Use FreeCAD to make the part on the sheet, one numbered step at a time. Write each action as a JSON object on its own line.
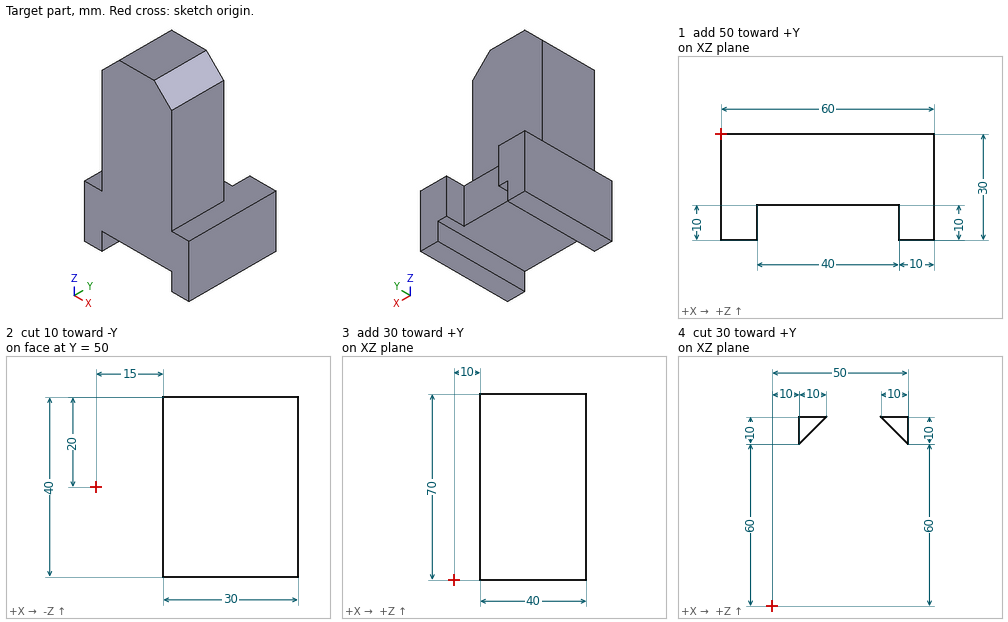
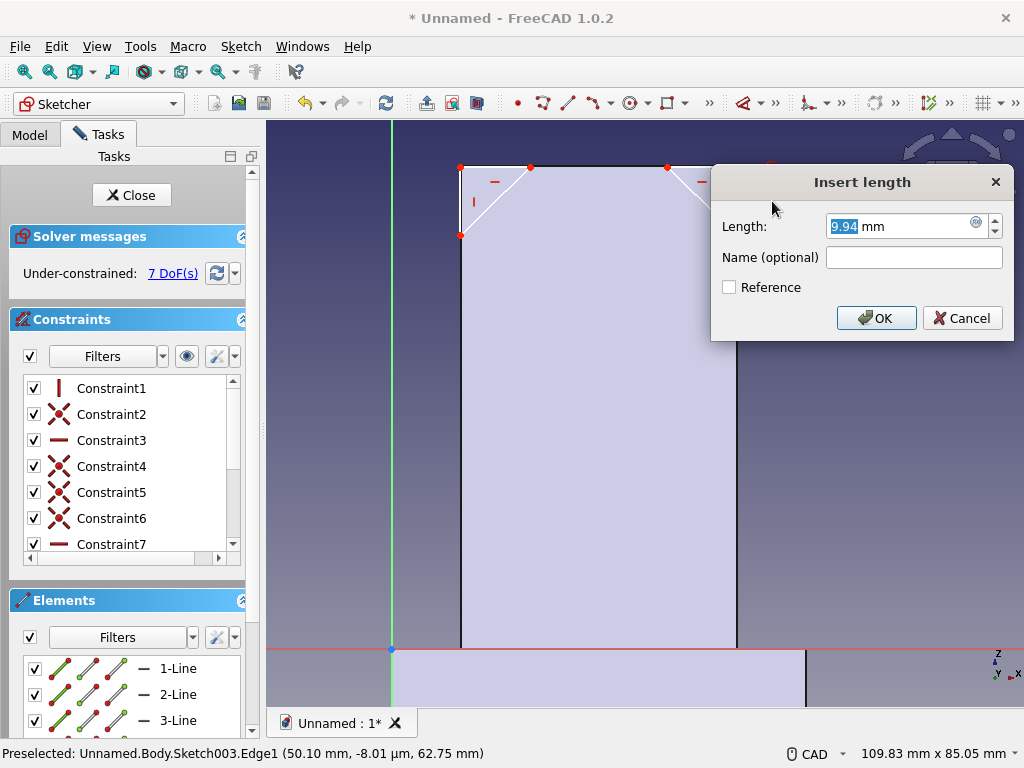
{"action": "type", "text": "10"}
{"action": "key", "text": "Return"}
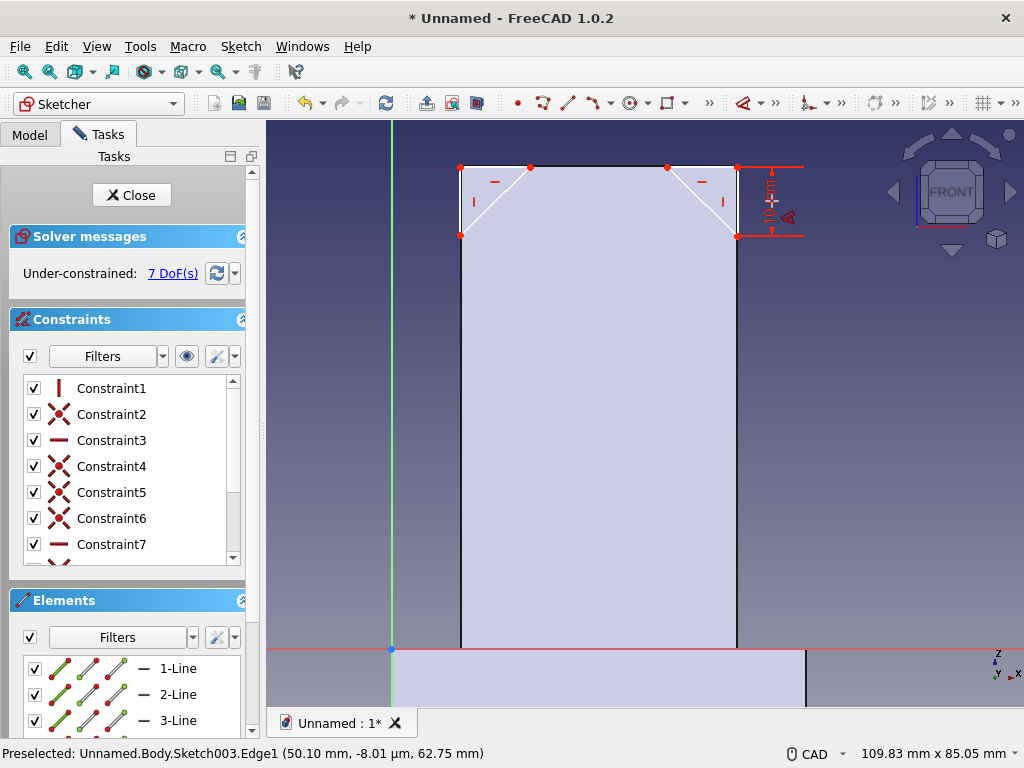
{"action": "left_click", "coordinate": [717, 167]}
{"action": "left_click", "coordinate": [678, 201]}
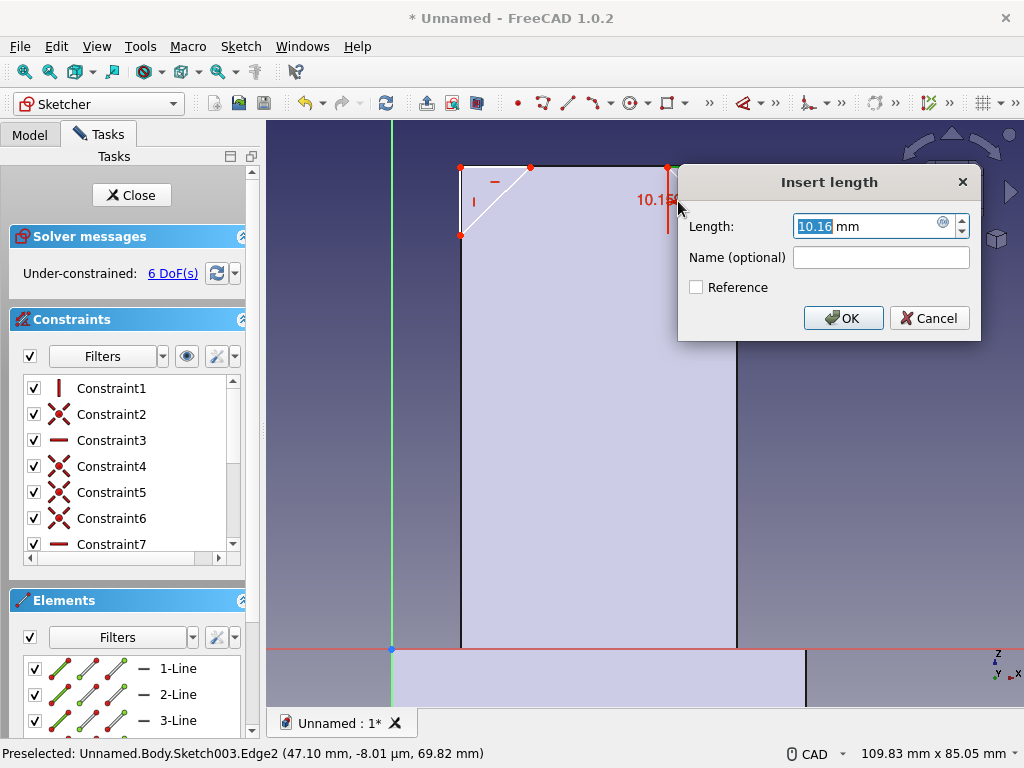
{"action": "type", "text": "10"}
{"action": "key", "text": "Return"}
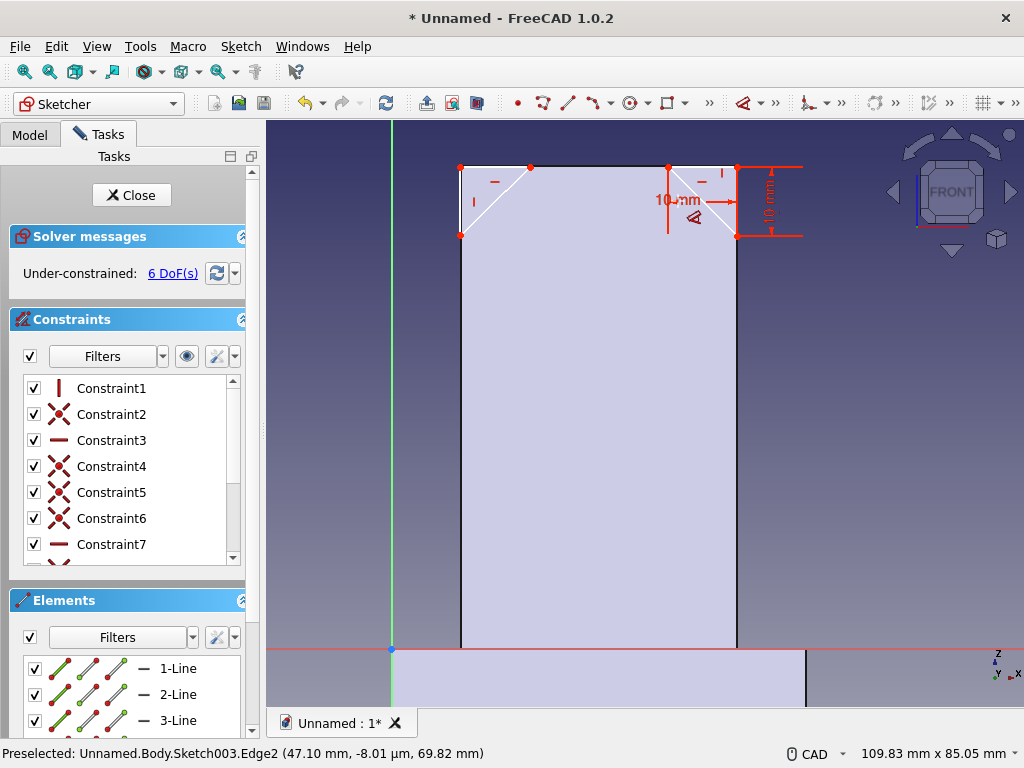
{"action": "left_click", "coordinate": [509, 167]}
{"action": "left_click", "coordinate": [520, 201]}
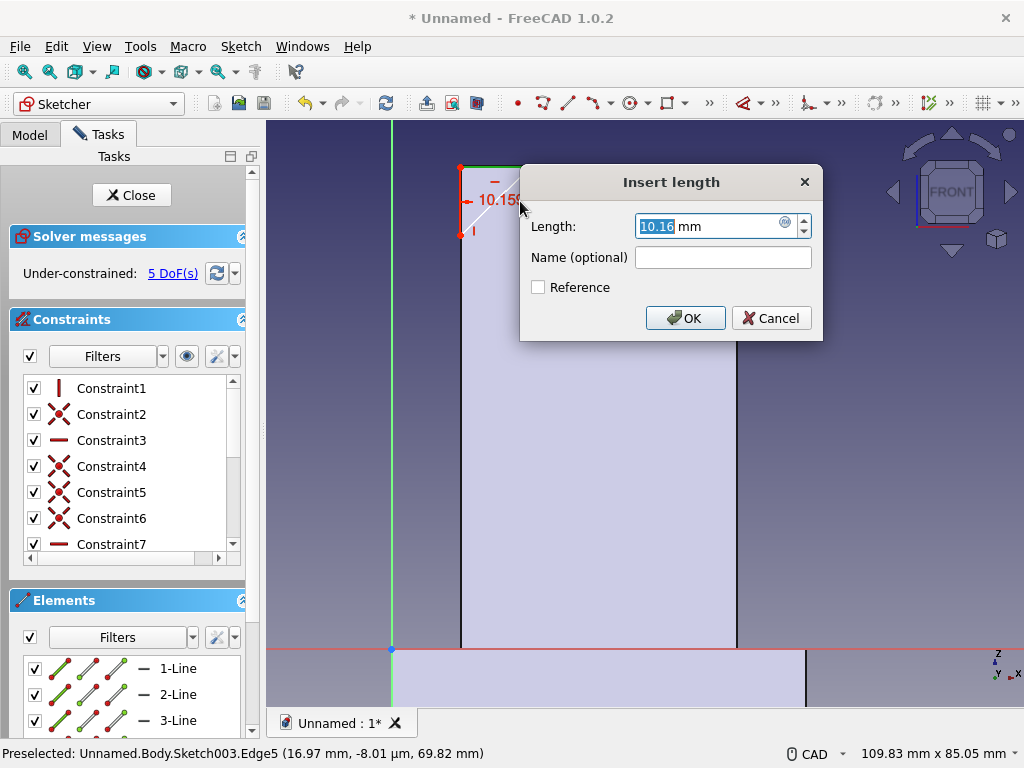
{"action": "type", "text": "10"}
{"action": "key", "text": "Return"}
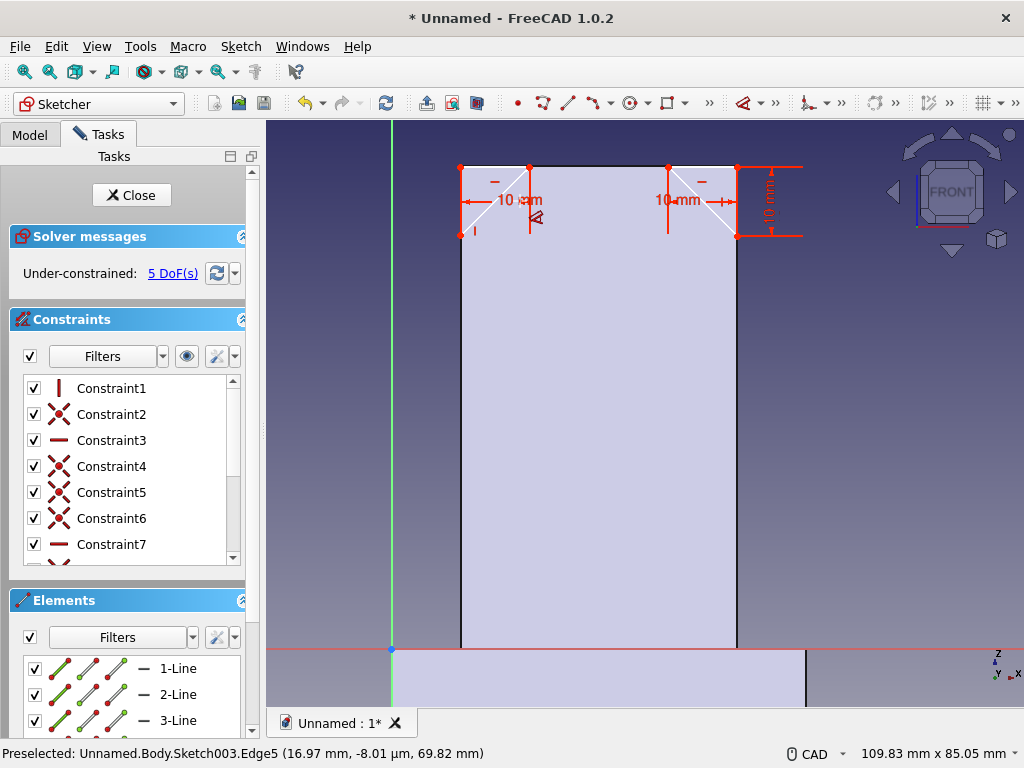
{"action": "left_click", "coordinate": [461, 188]}
{"action": "left_click", "coordinate": [427, 201]}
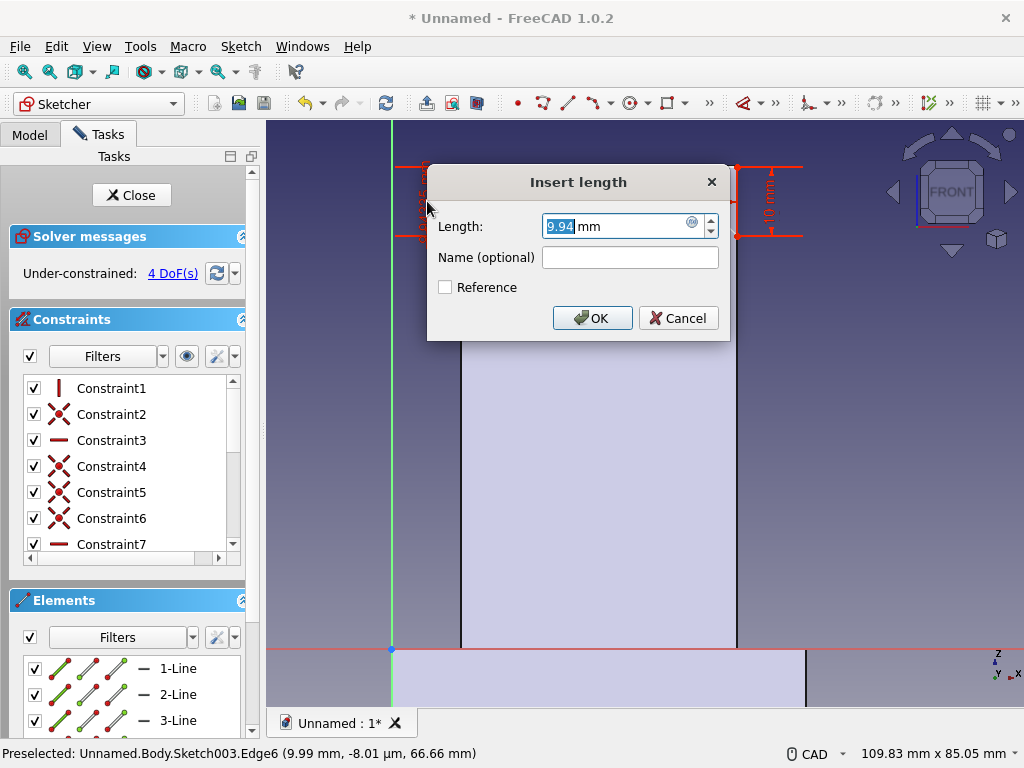
{"action": "type", "text": "10"}
{"action": "key", "text": "Return"}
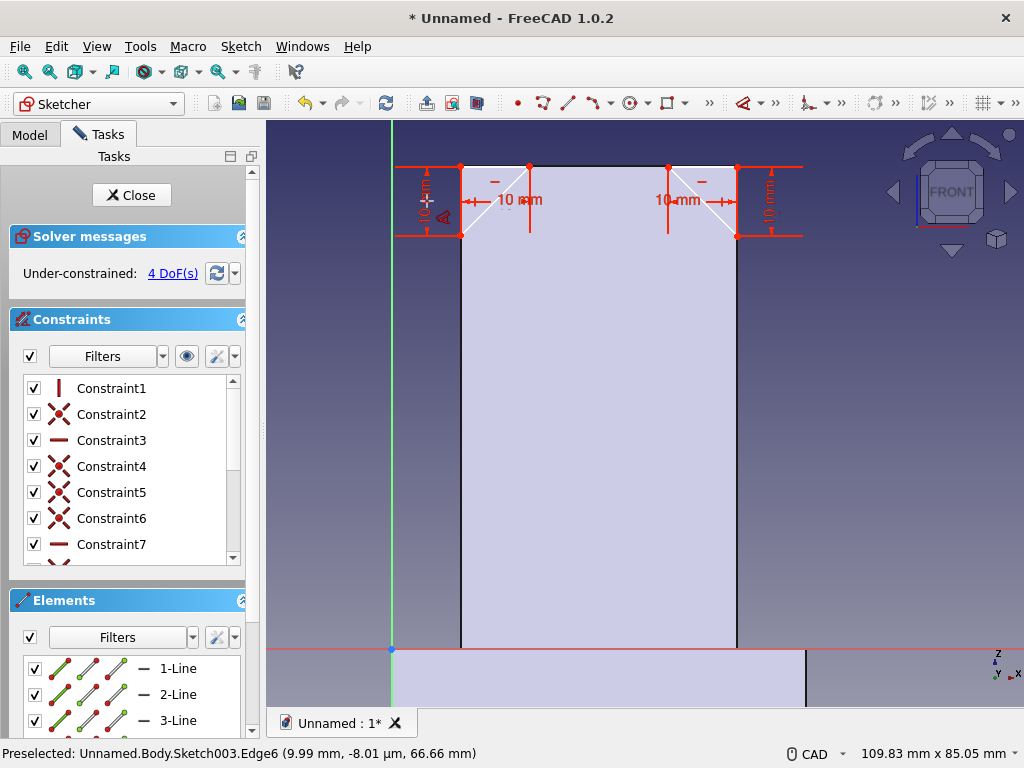
{"action": "left_click", "coordinate": [737, 236]}
{"action": "left_click", "coordinate": [565, 178]}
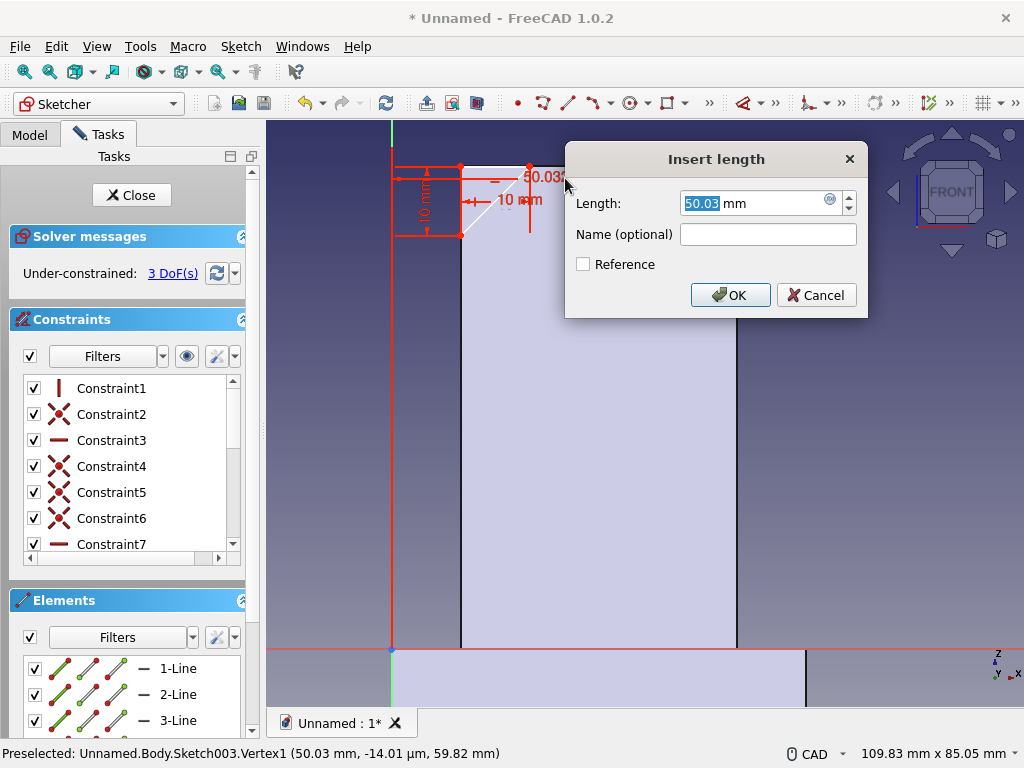
{"action": "type", "text": "50"}
{"action": "key", "text": "Return"}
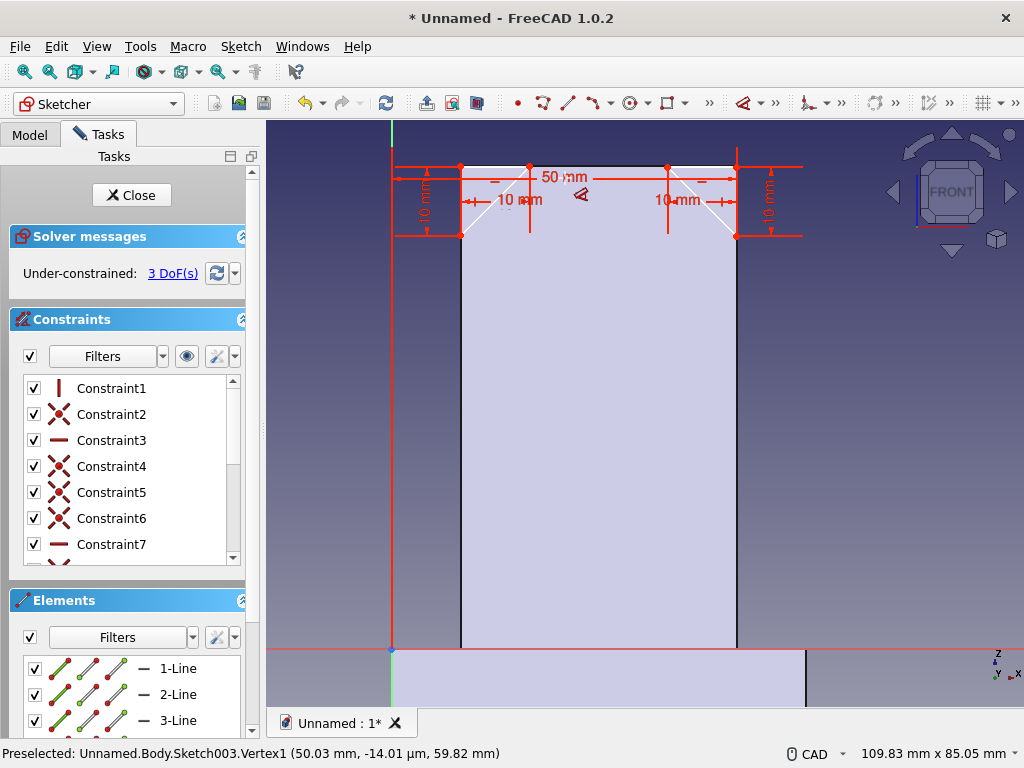
{"action": "left_click", "coordinate": [737, 236]}
{"action": "left_click", "coordinate": [771, 443]}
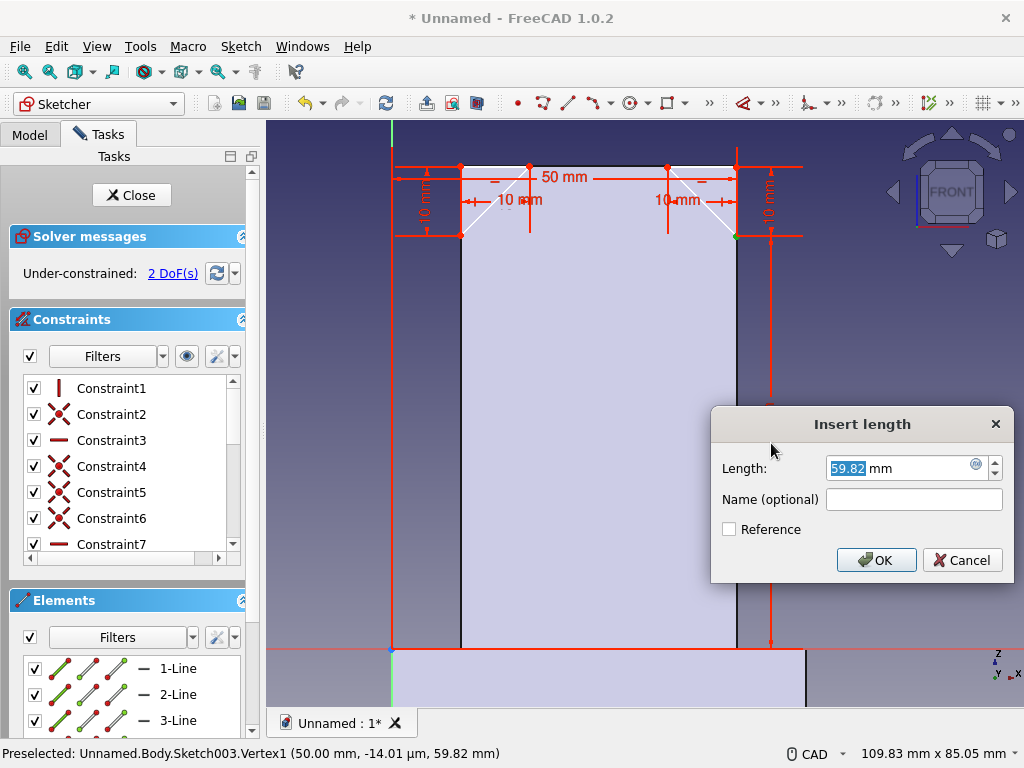
{"action": "type", "text": "60"}
{"action": "key", "text": "Return"}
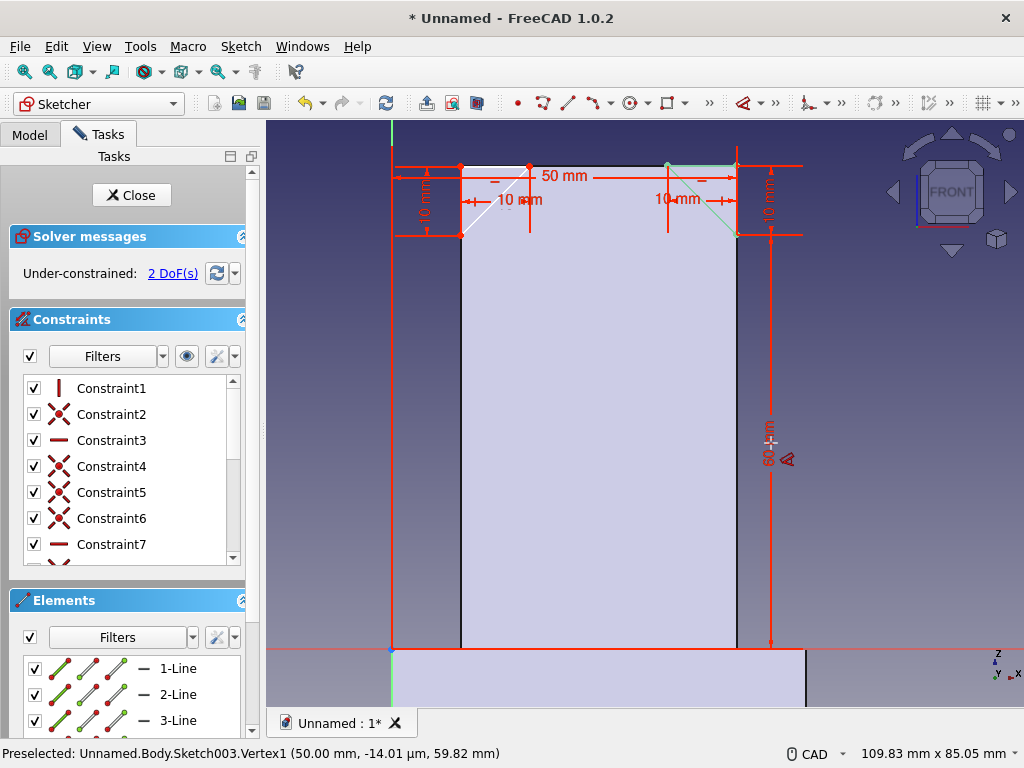
{"action": "left_click", "coordinate": [461, 236]}
{"action": "left_click", "coordinate": [426, 178]}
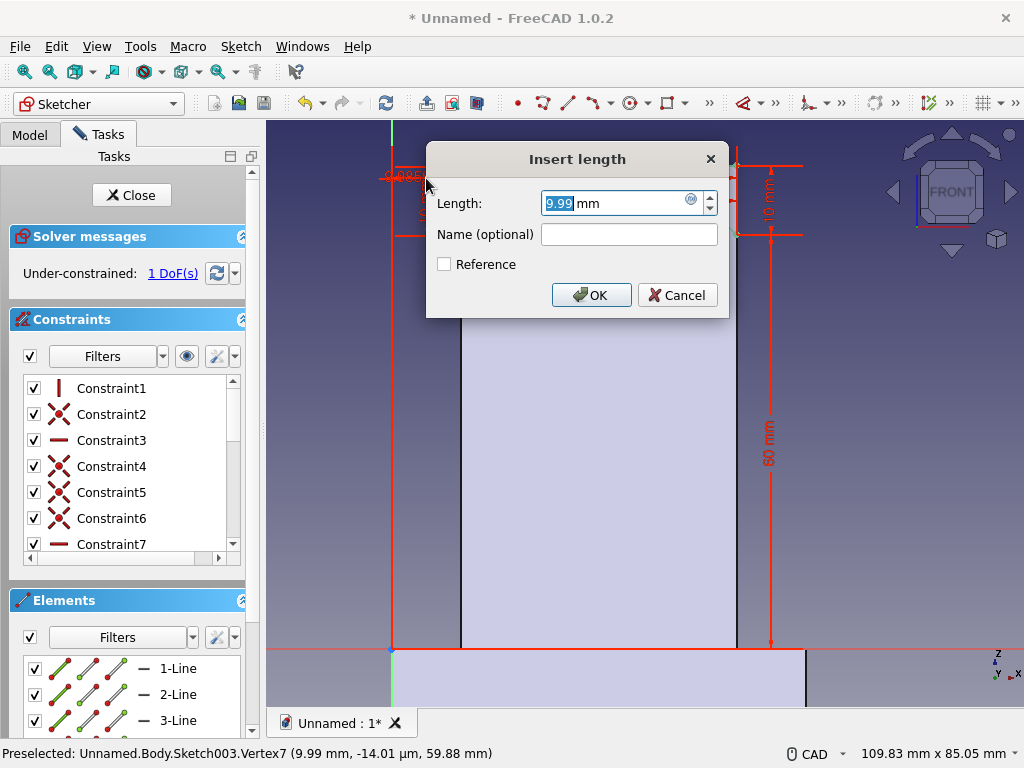
{"action": "type", "text": "10"}
{"action": "key", "text": "Return"}